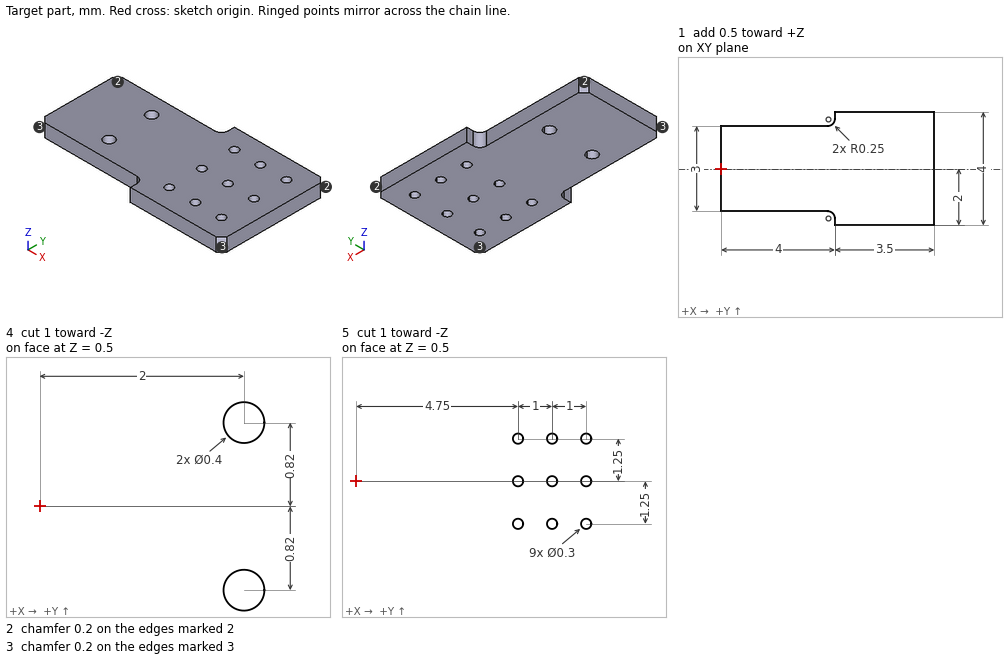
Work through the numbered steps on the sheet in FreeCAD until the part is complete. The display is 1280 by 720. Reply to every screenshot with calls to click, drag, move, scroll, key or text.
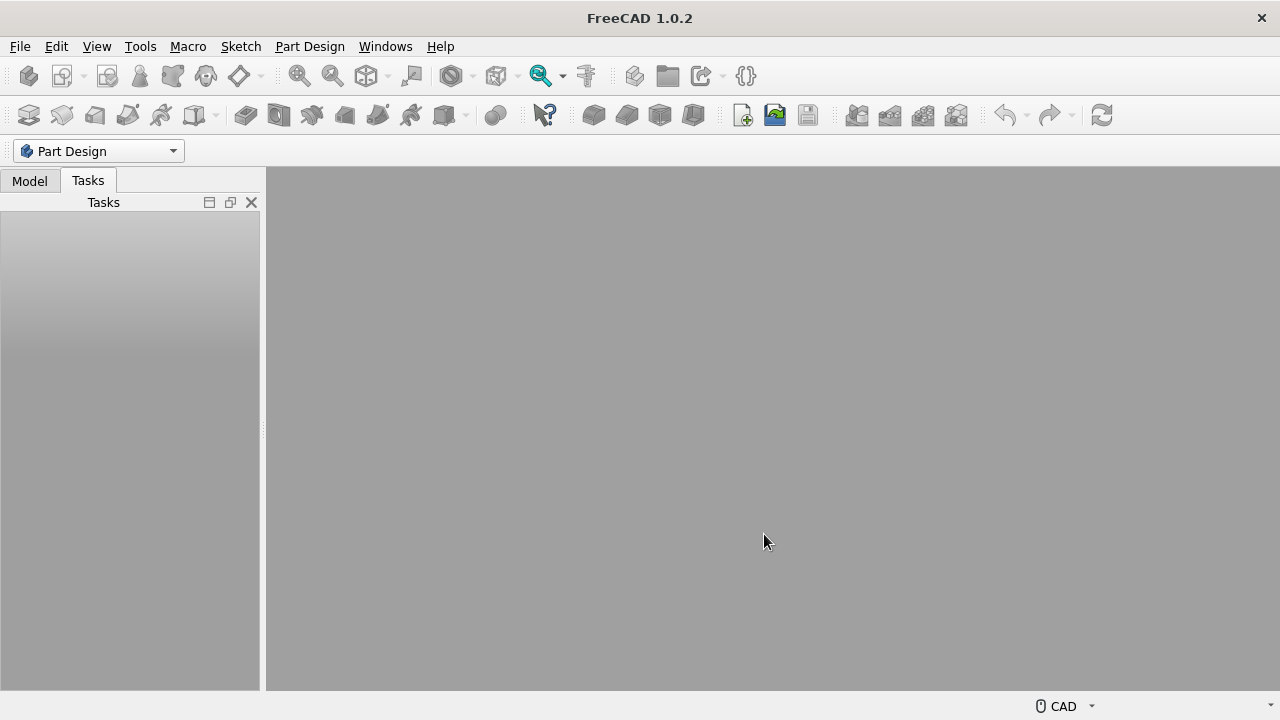
key(ctrl+n)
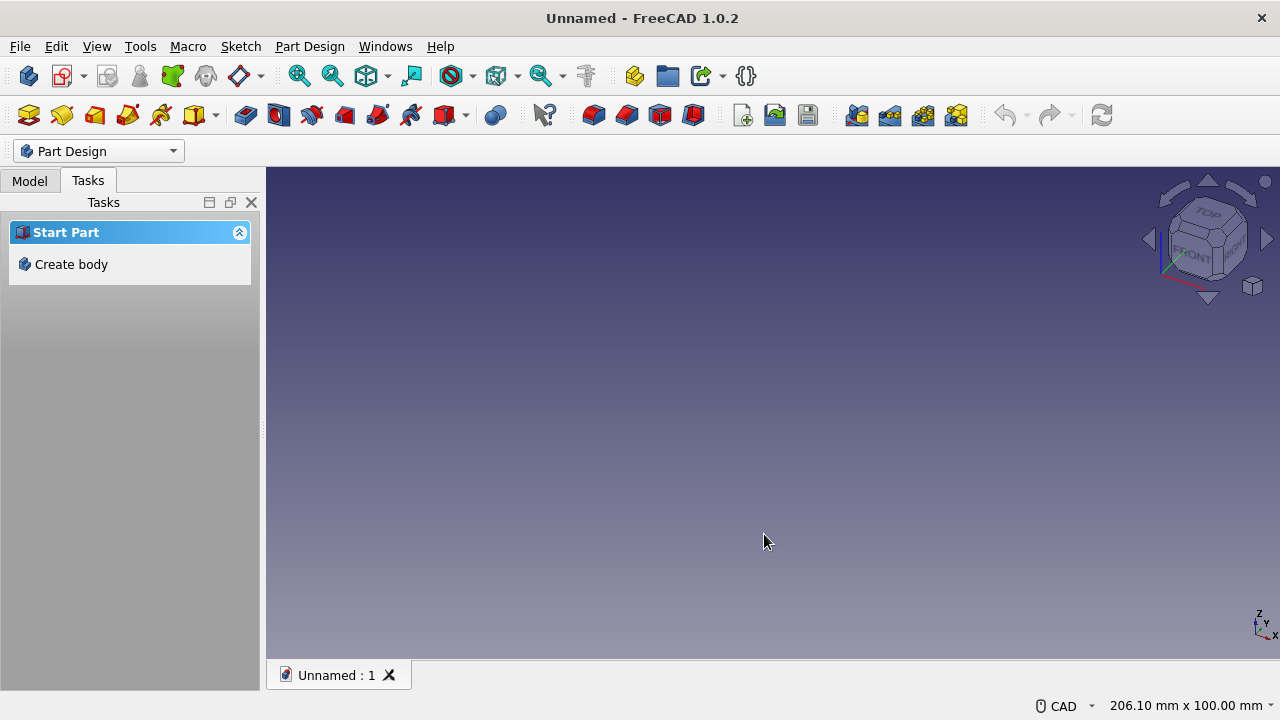
click(62, 76)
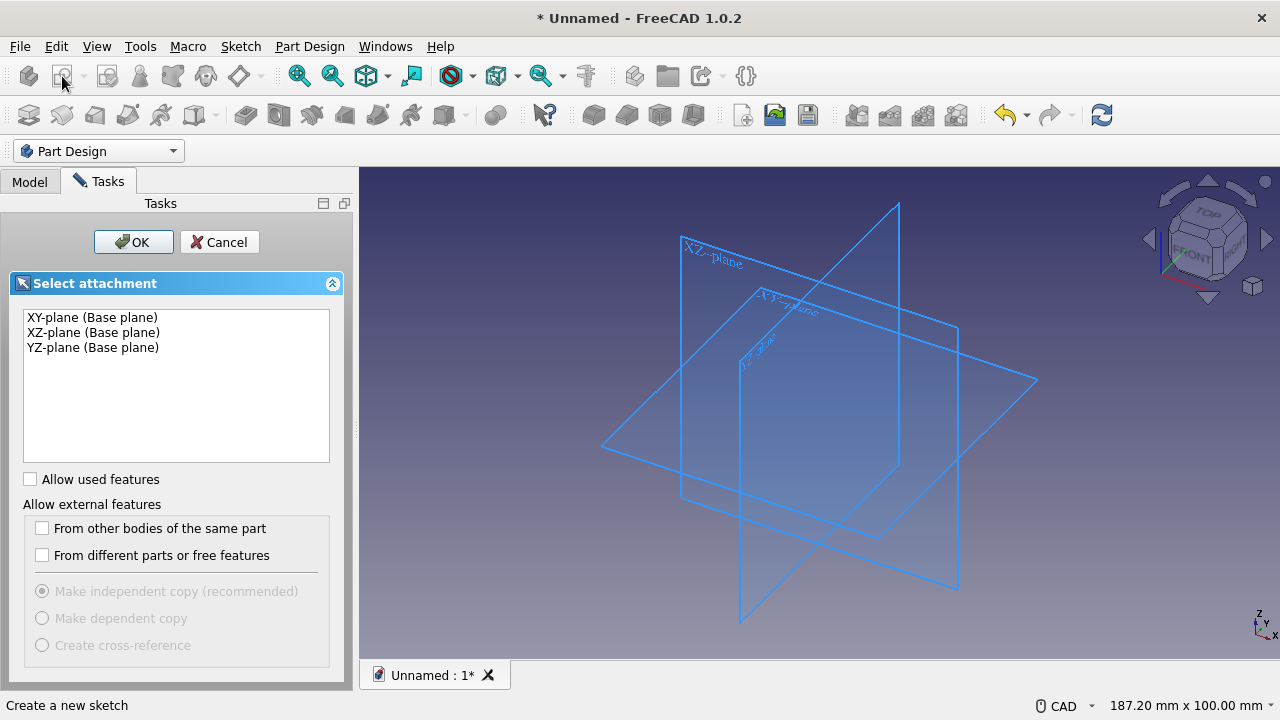
click(84, 318)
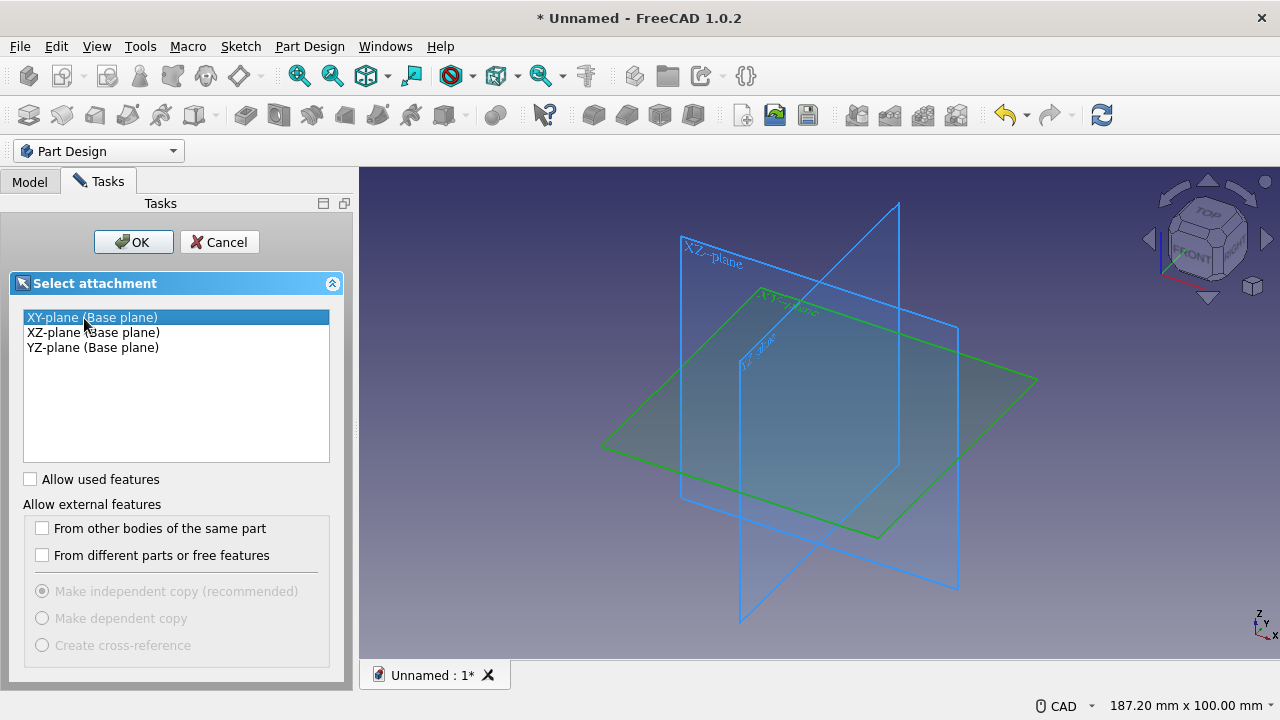
click(134, 242)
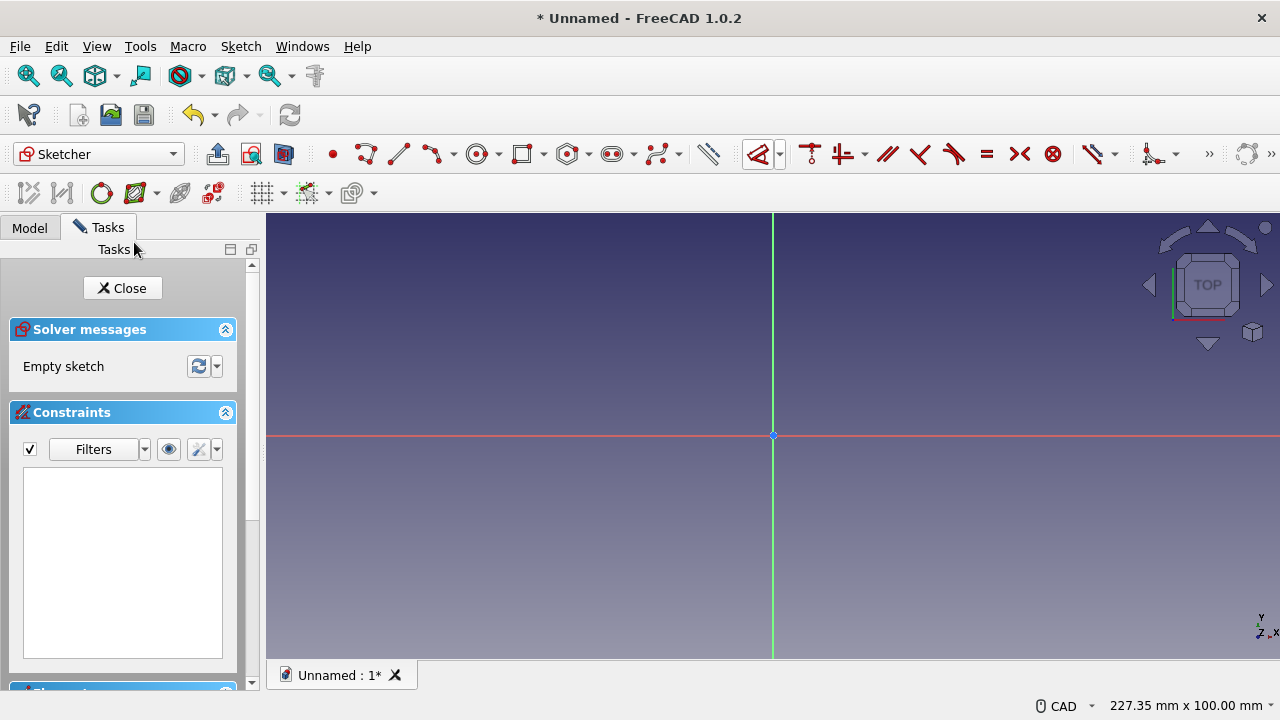
scroll(795, 436, up, 14)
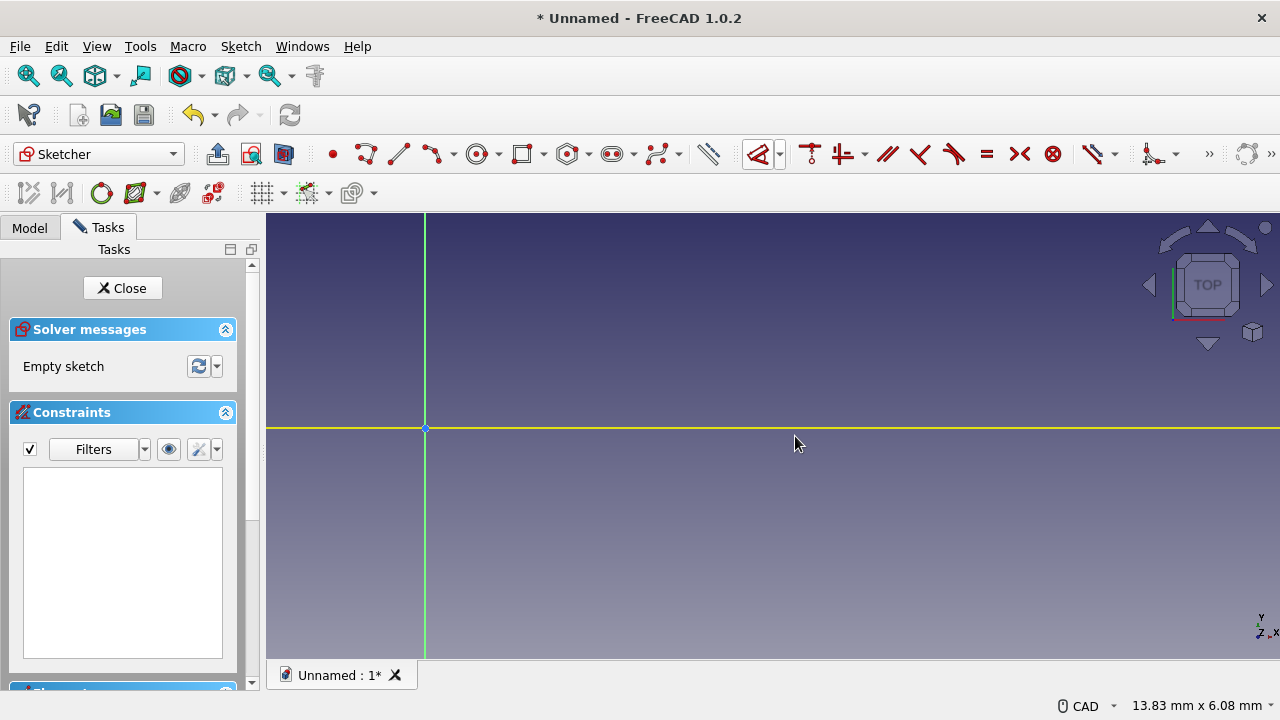
key(g)
key(m)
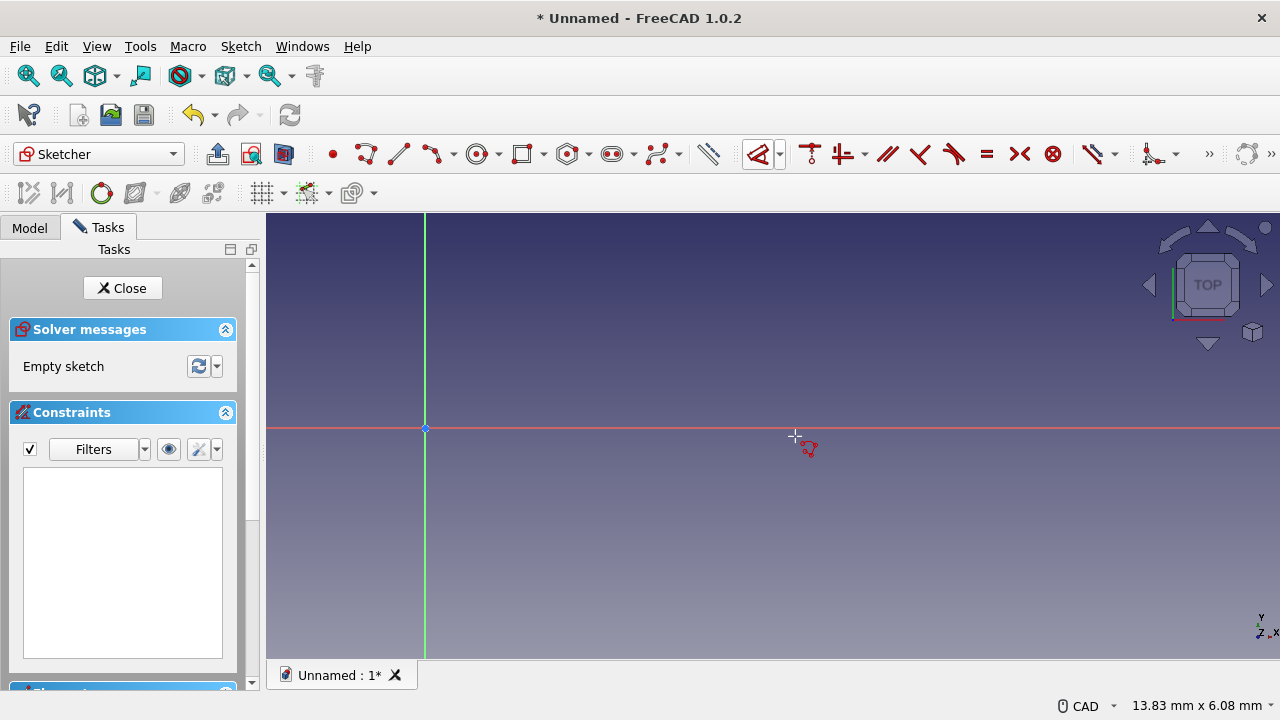
click(700, 318)
click(425, 318)
click(434, 538)
click(700, 538)
right_click(700, 538)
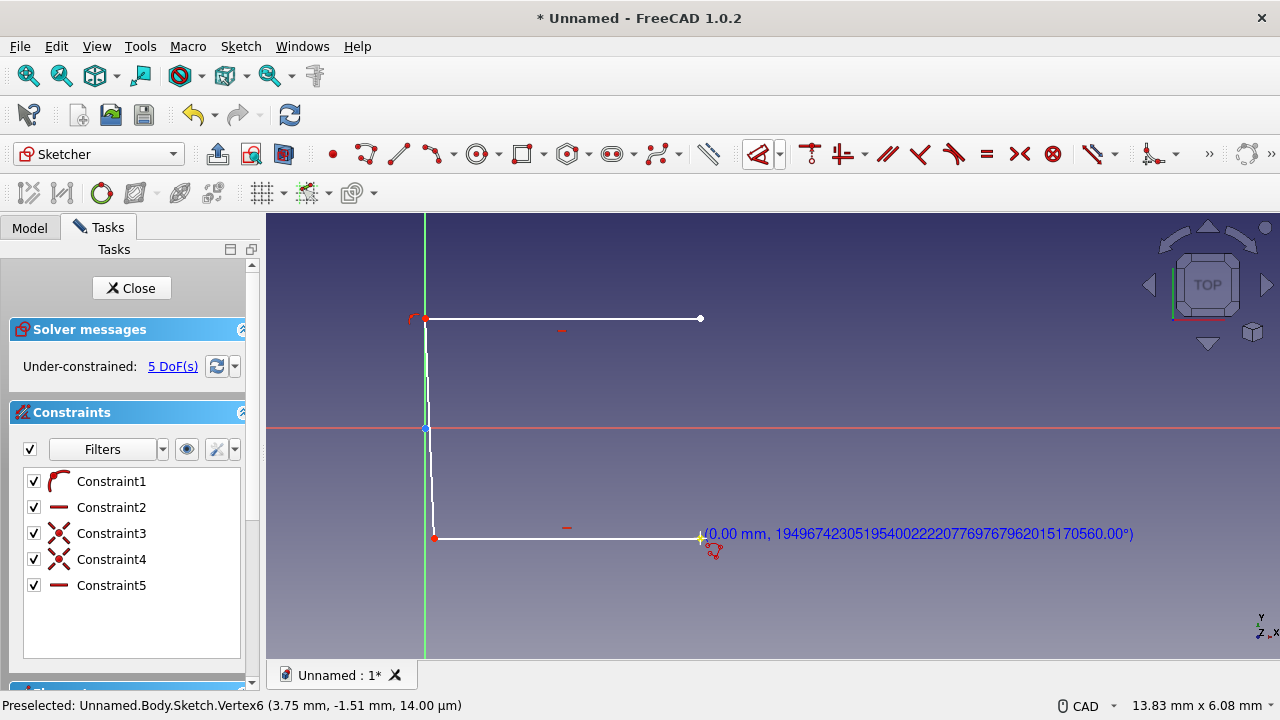
click(719, 557)
click(719, 575)
click(975, 575)
click(975, 282)
click(719, 282)
click(719, 300)
right_click(719, 300)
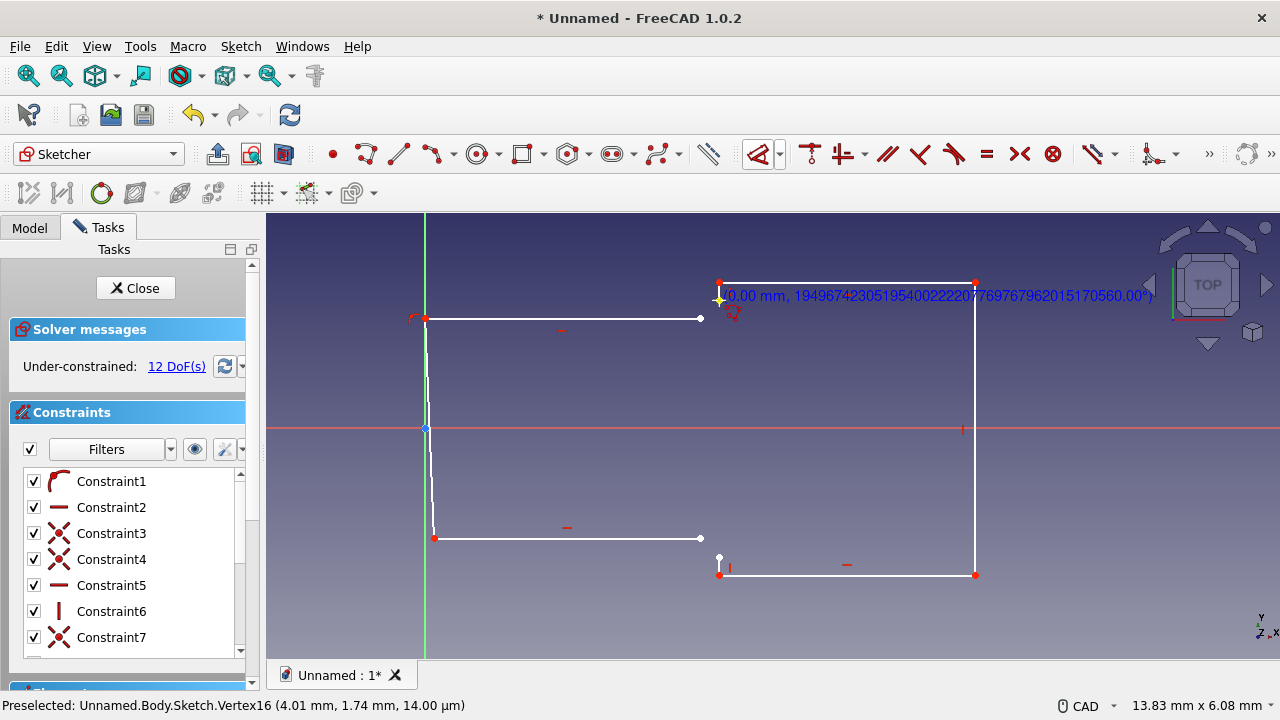
click(432, 154)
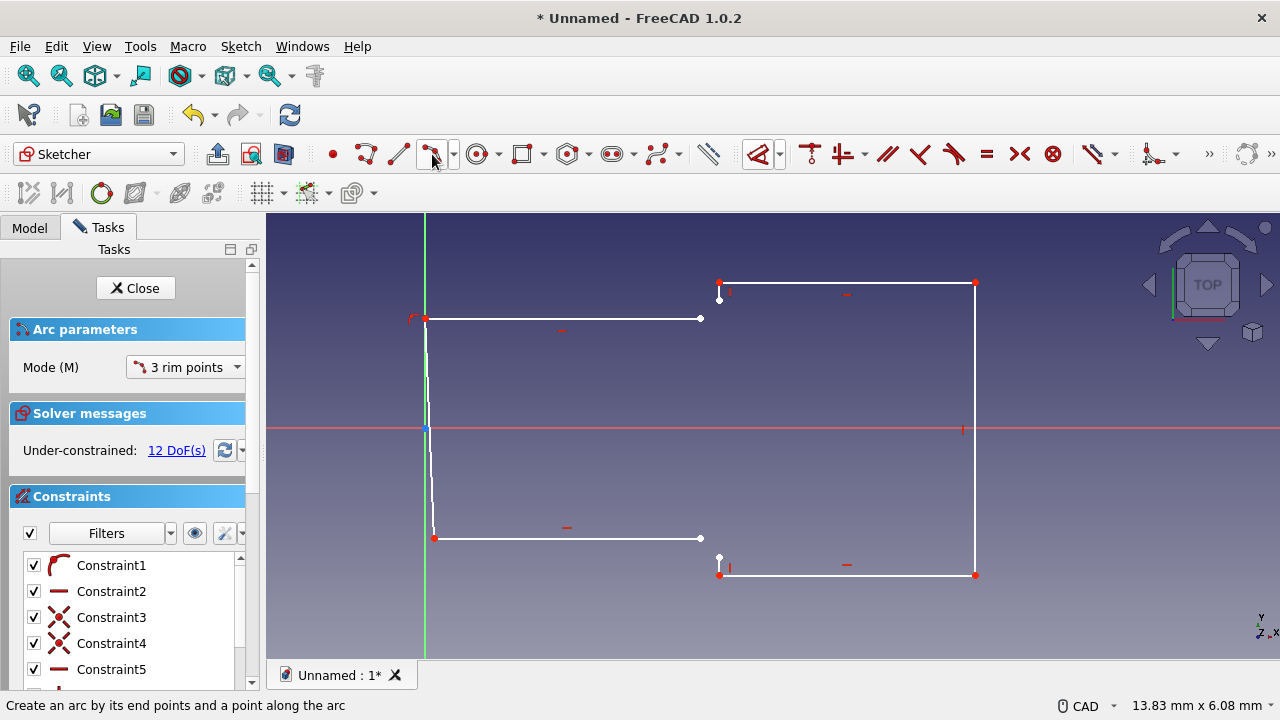
click(700, 539)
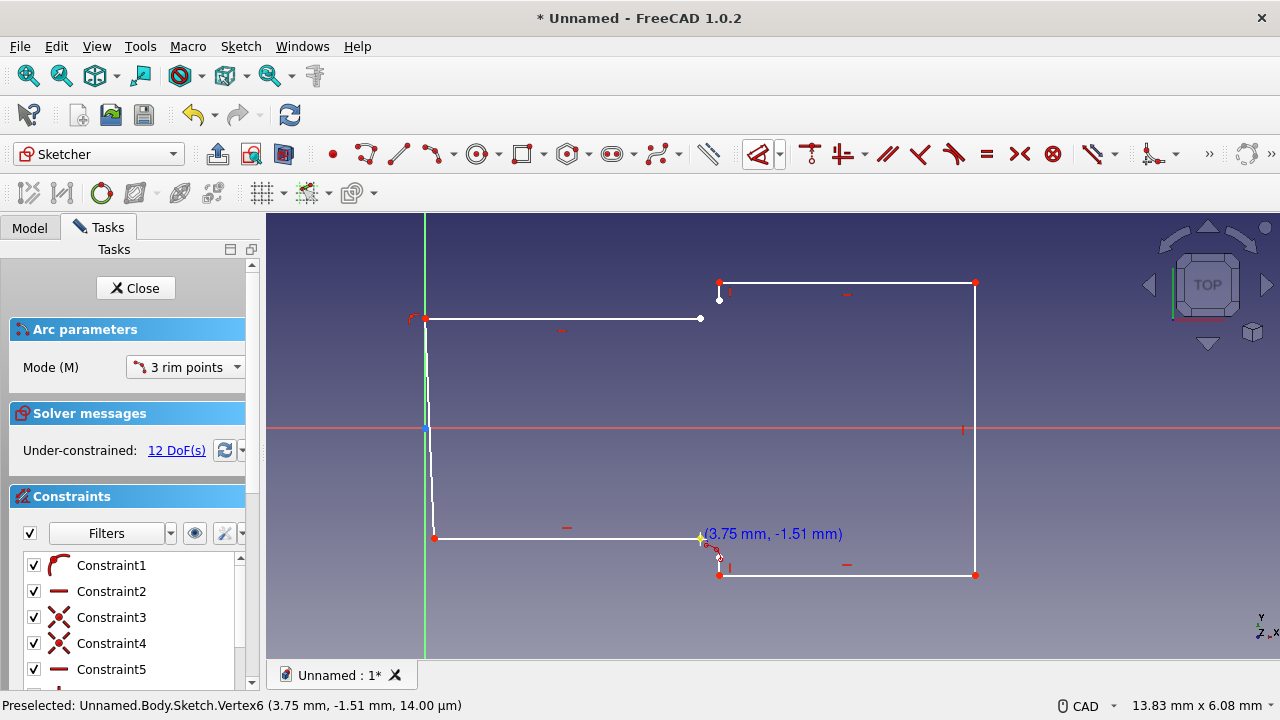
scroll(719, 557, up, 3)